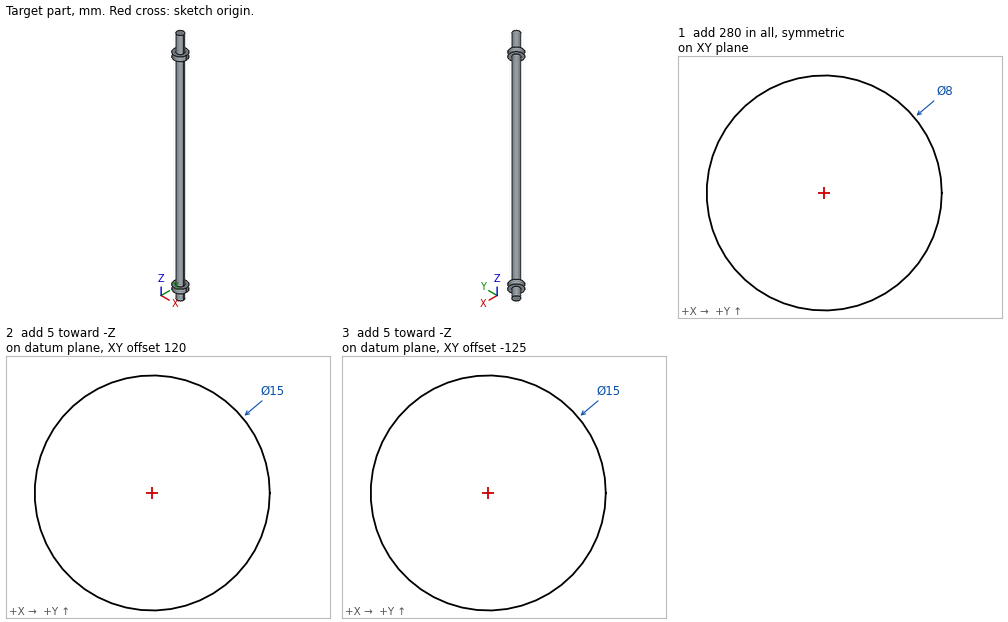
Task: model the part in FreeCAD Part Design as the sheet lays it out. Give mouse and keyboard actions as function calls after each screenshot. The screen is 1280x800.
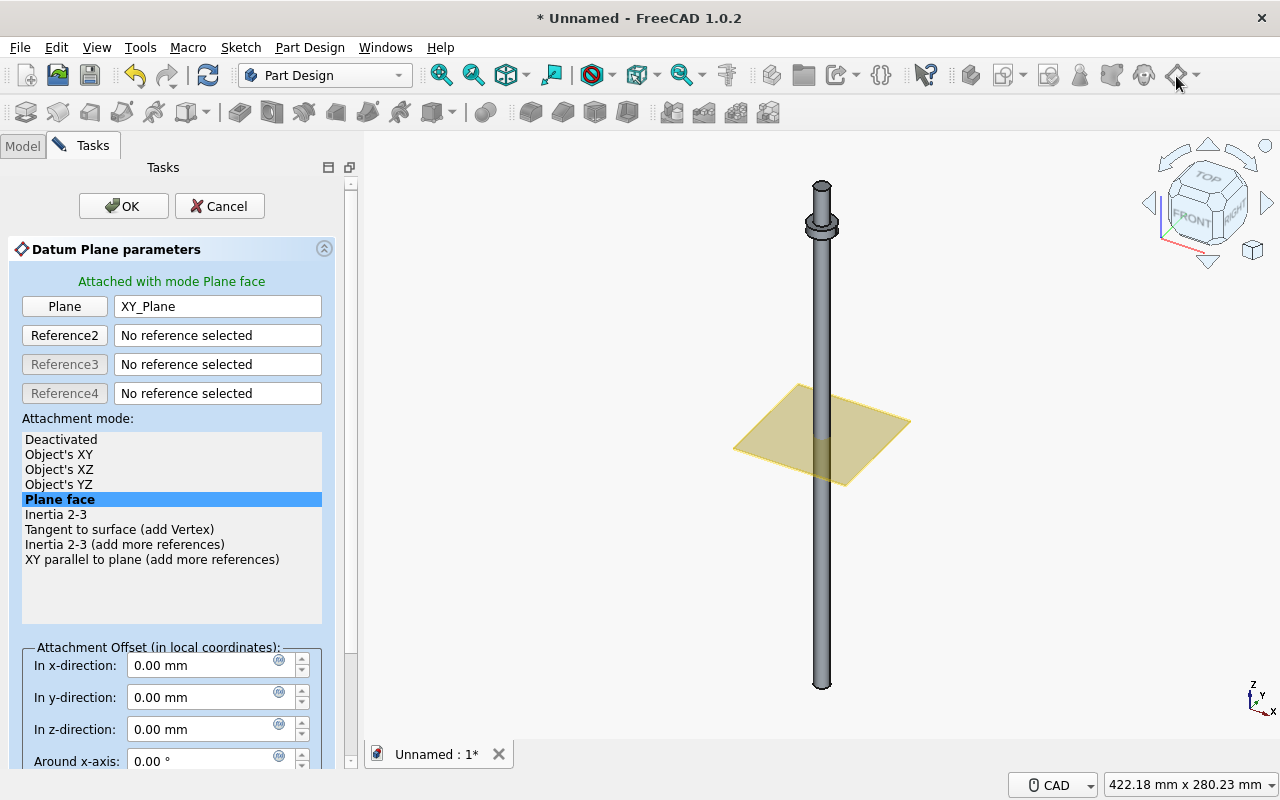
triple_click(210, 729)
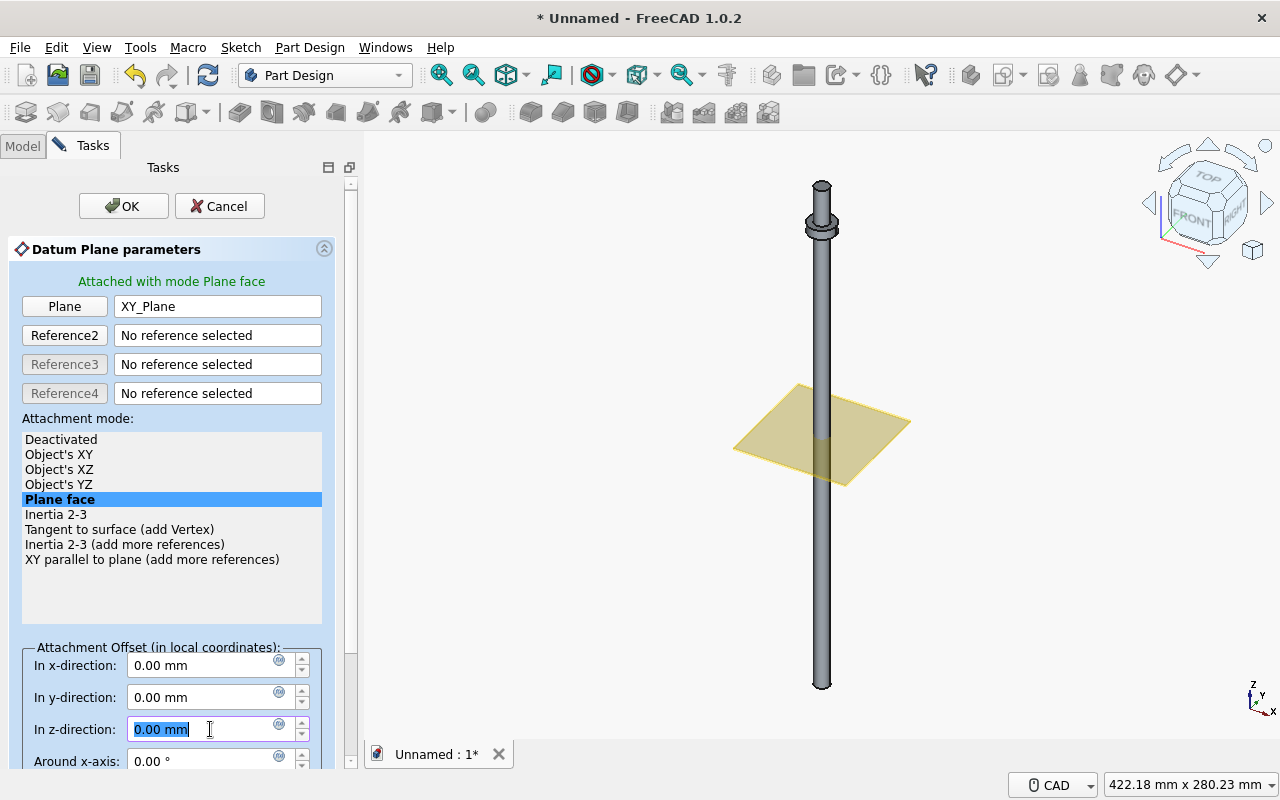
text(-125)
key(Tab)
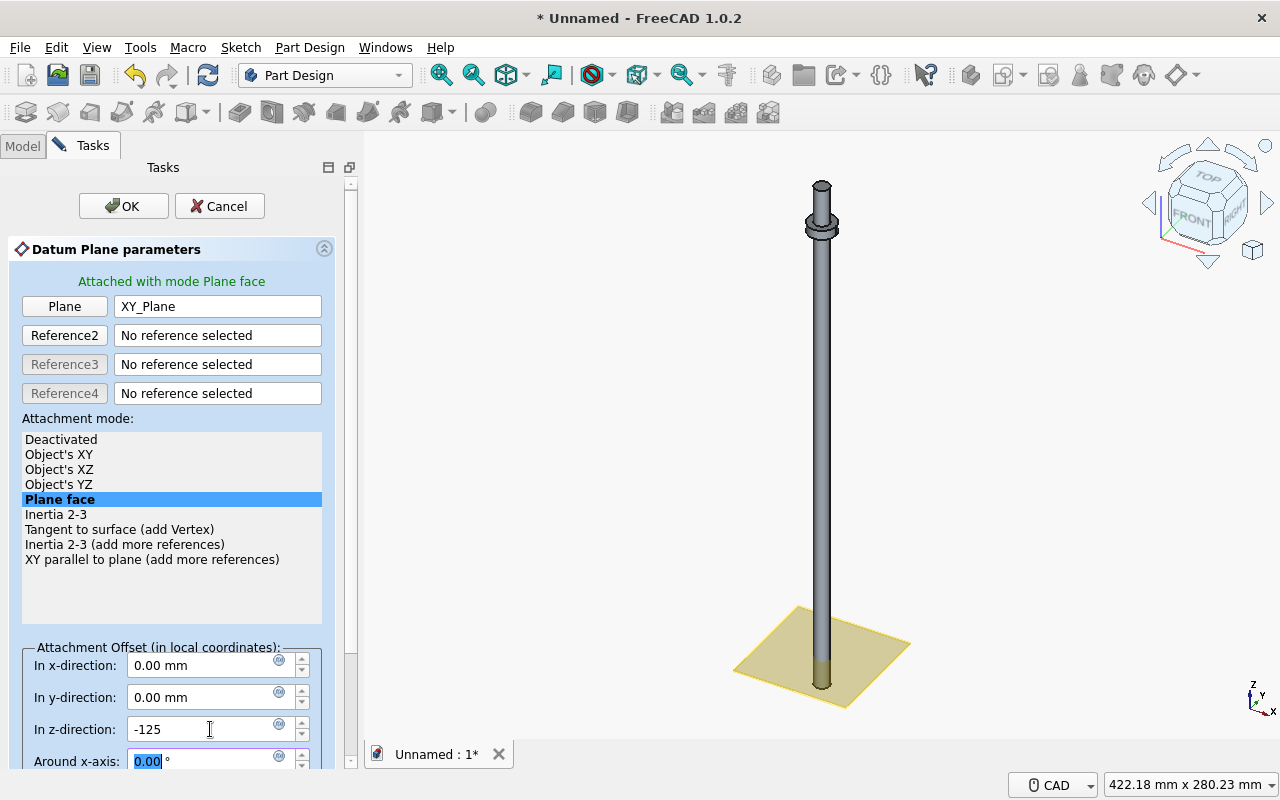
click(124, 206)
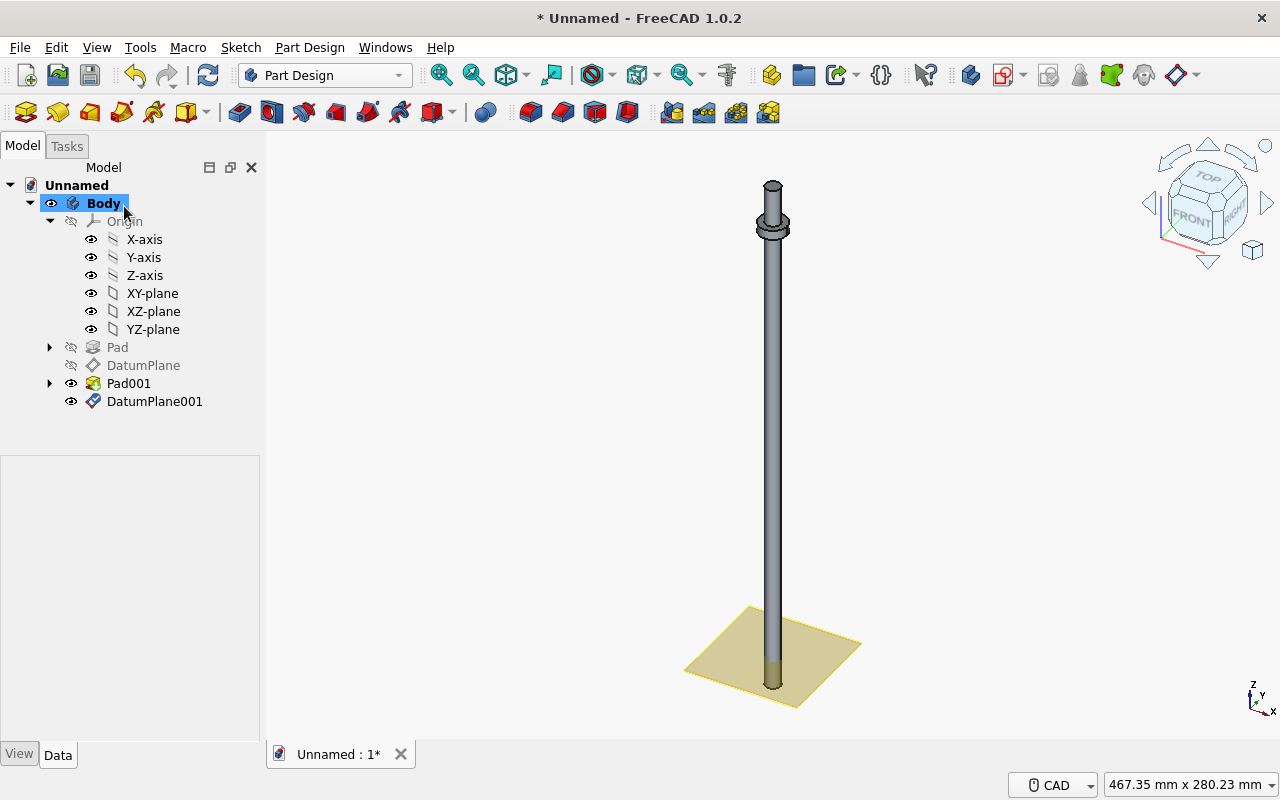
click(116, 401)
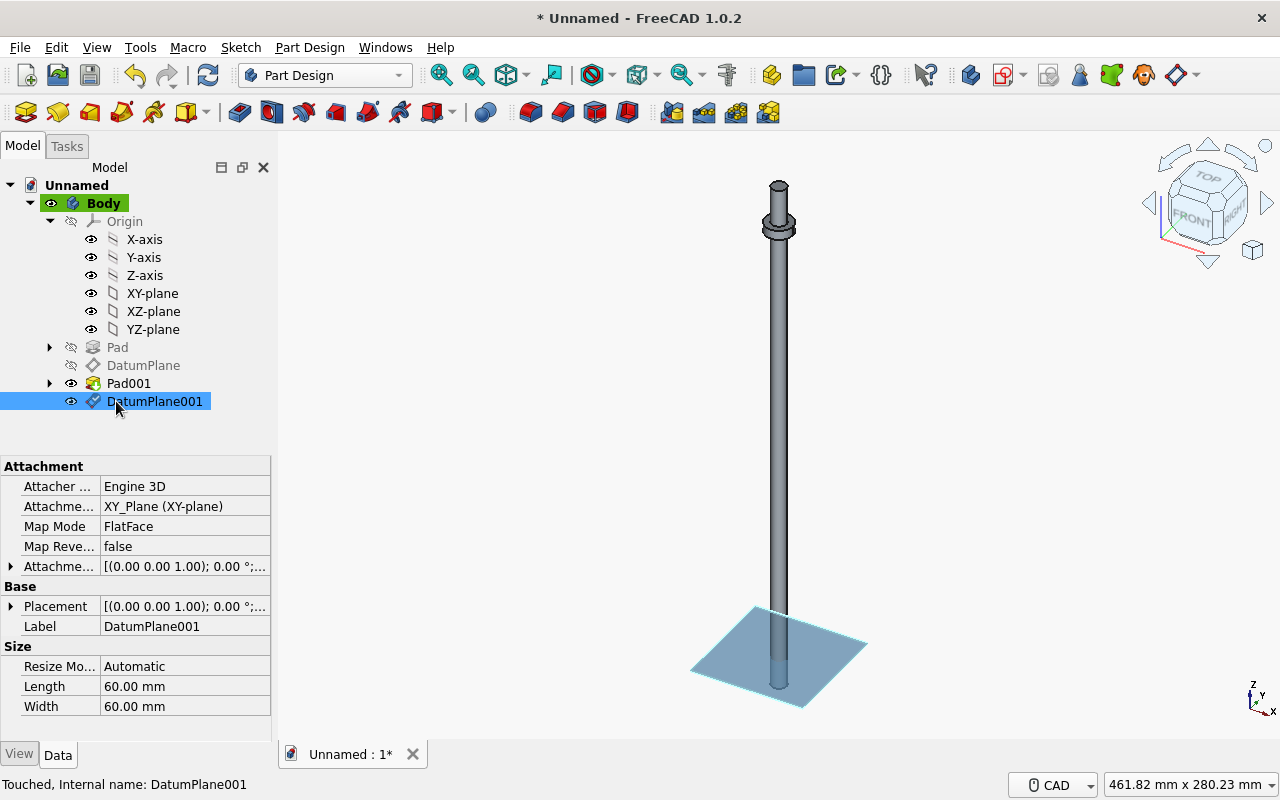
click(1004, 76)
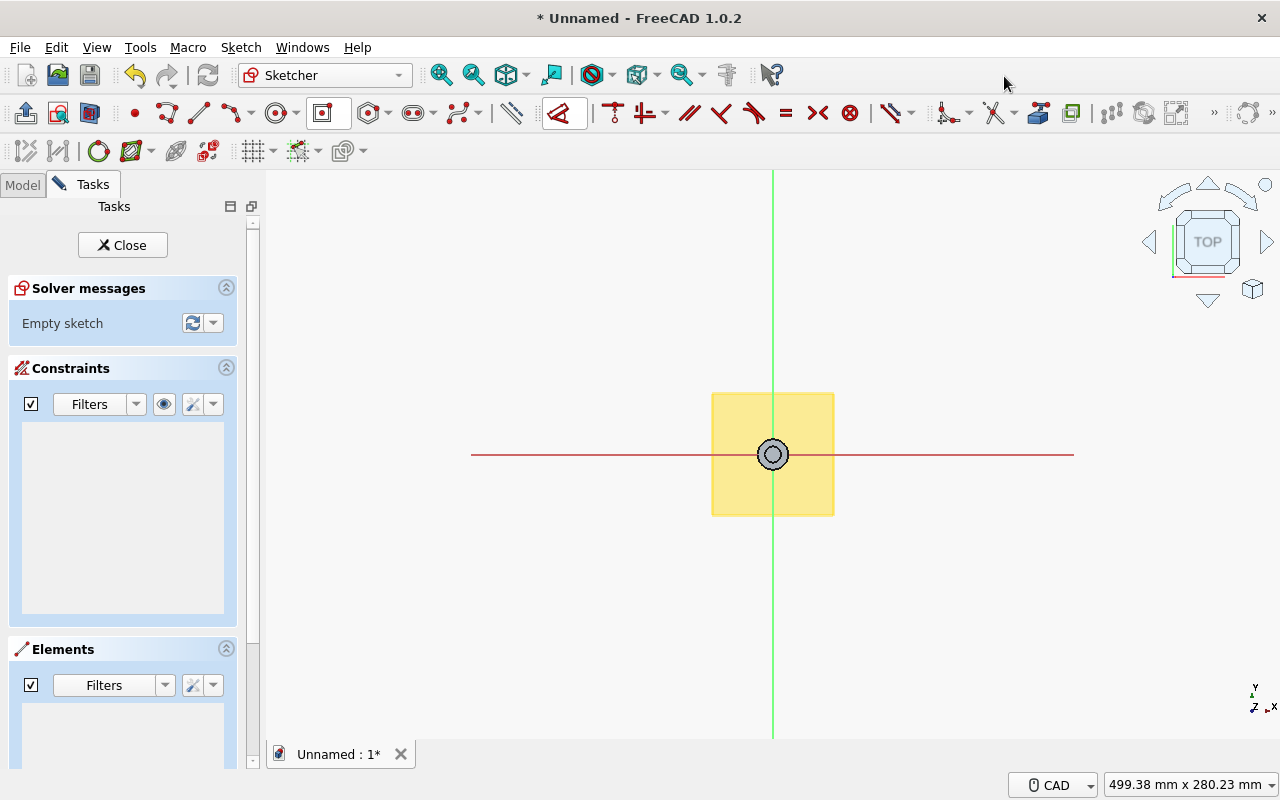
key(q)
key(s)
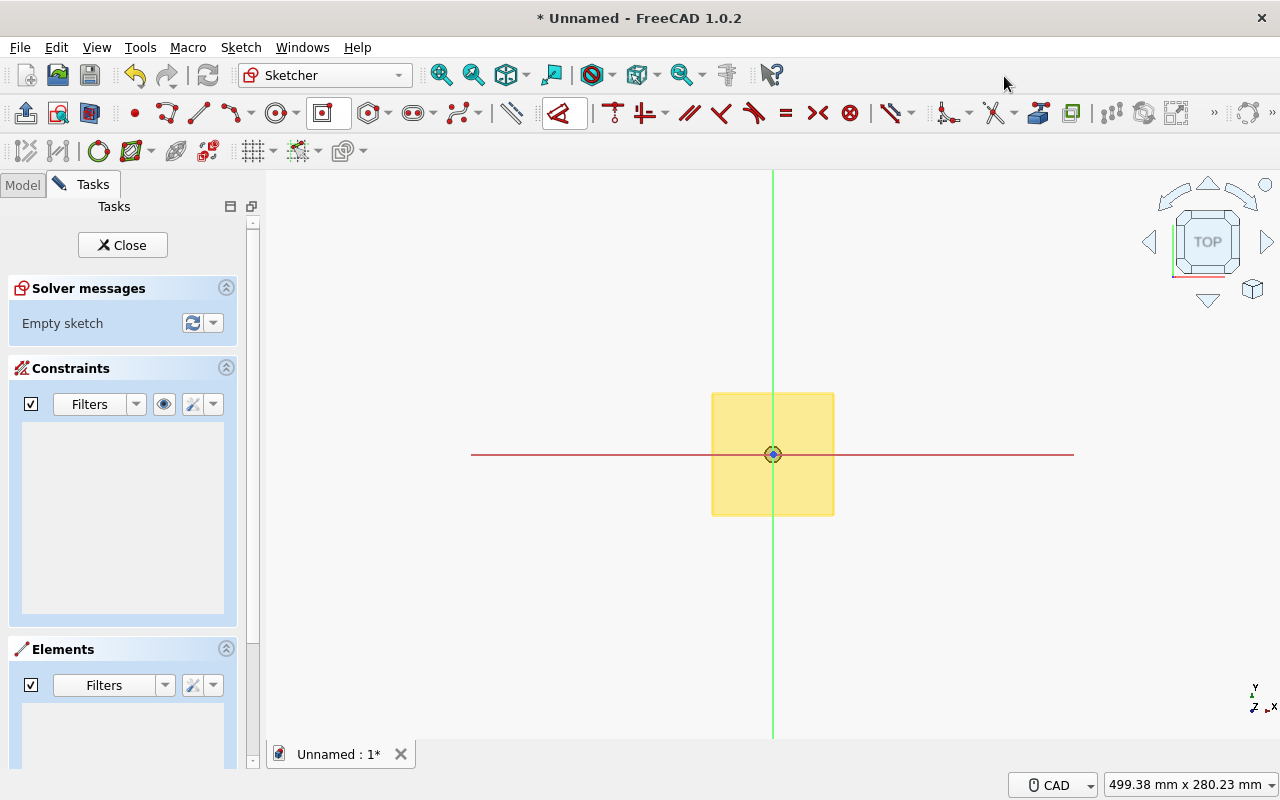
scroll(780, 455, up, 12)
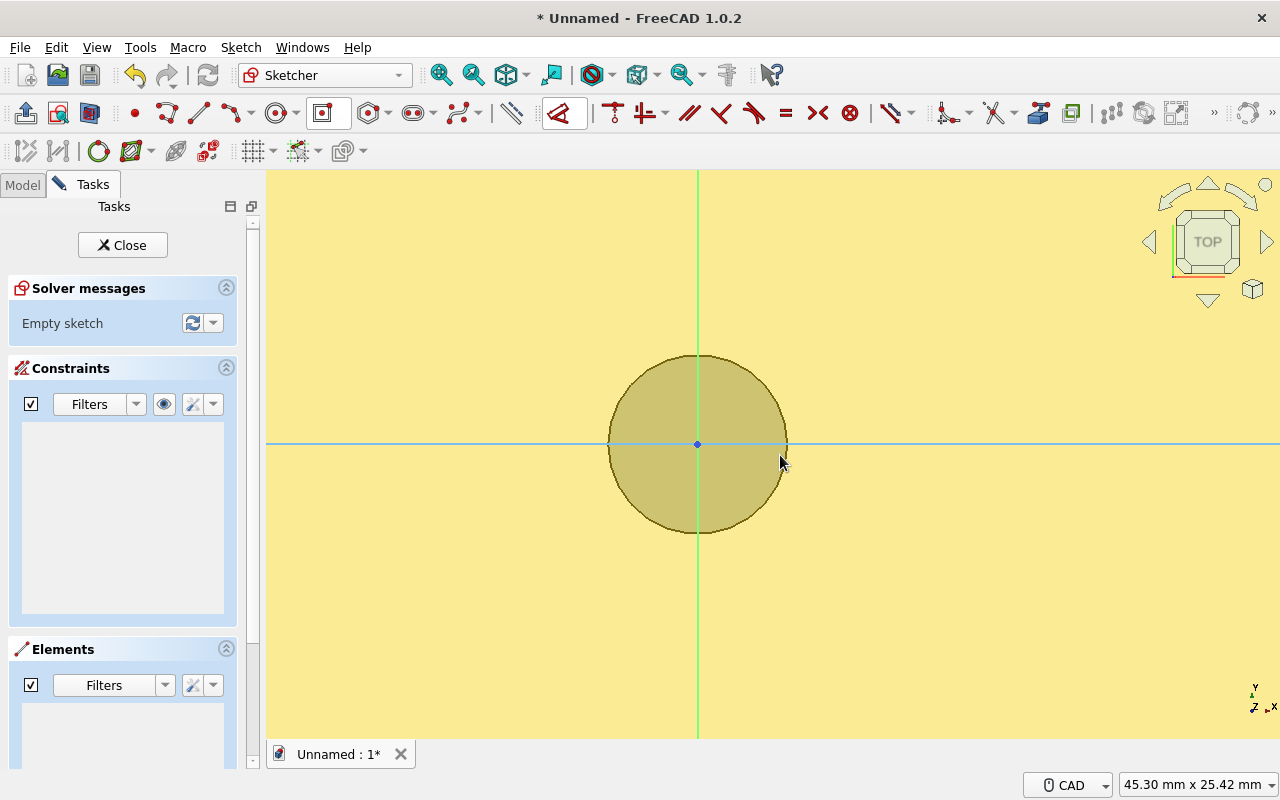
key(g)
key(c)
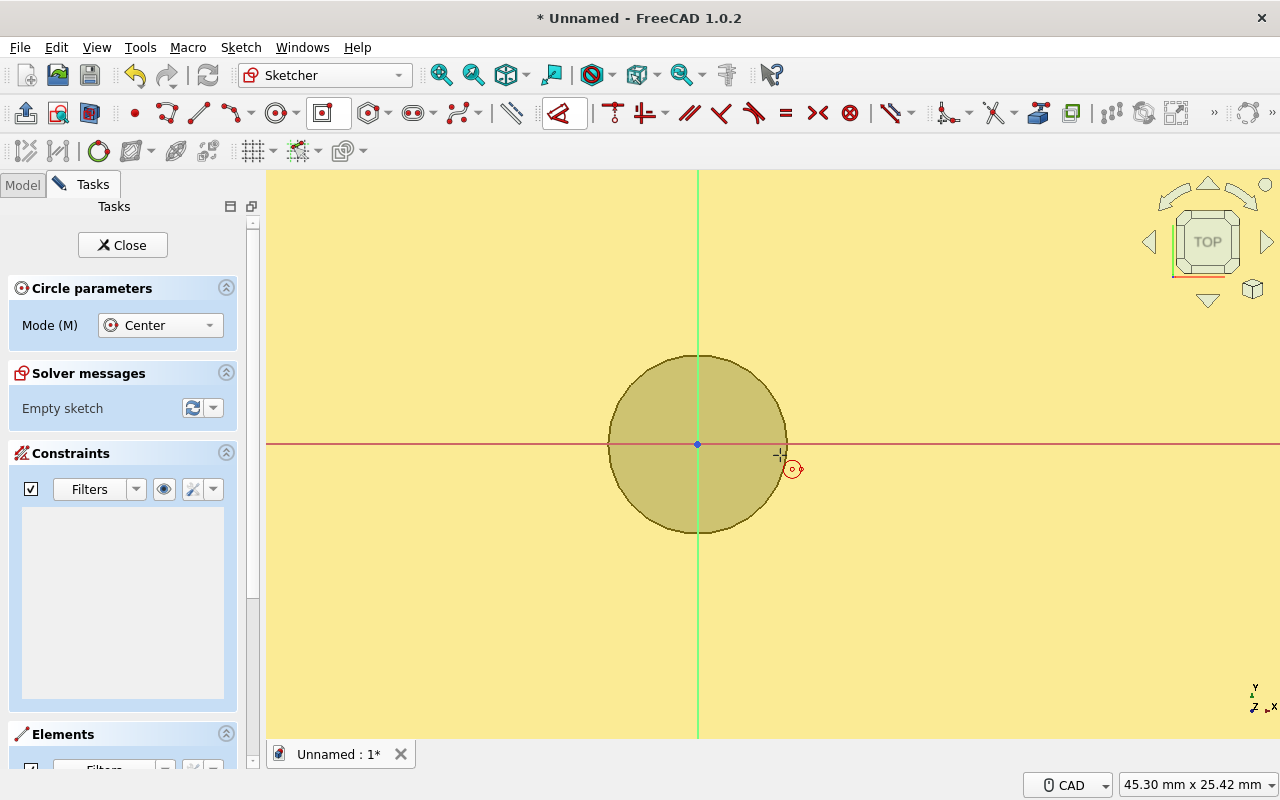
click(698, 444)
click(816, 326)
key(Escape)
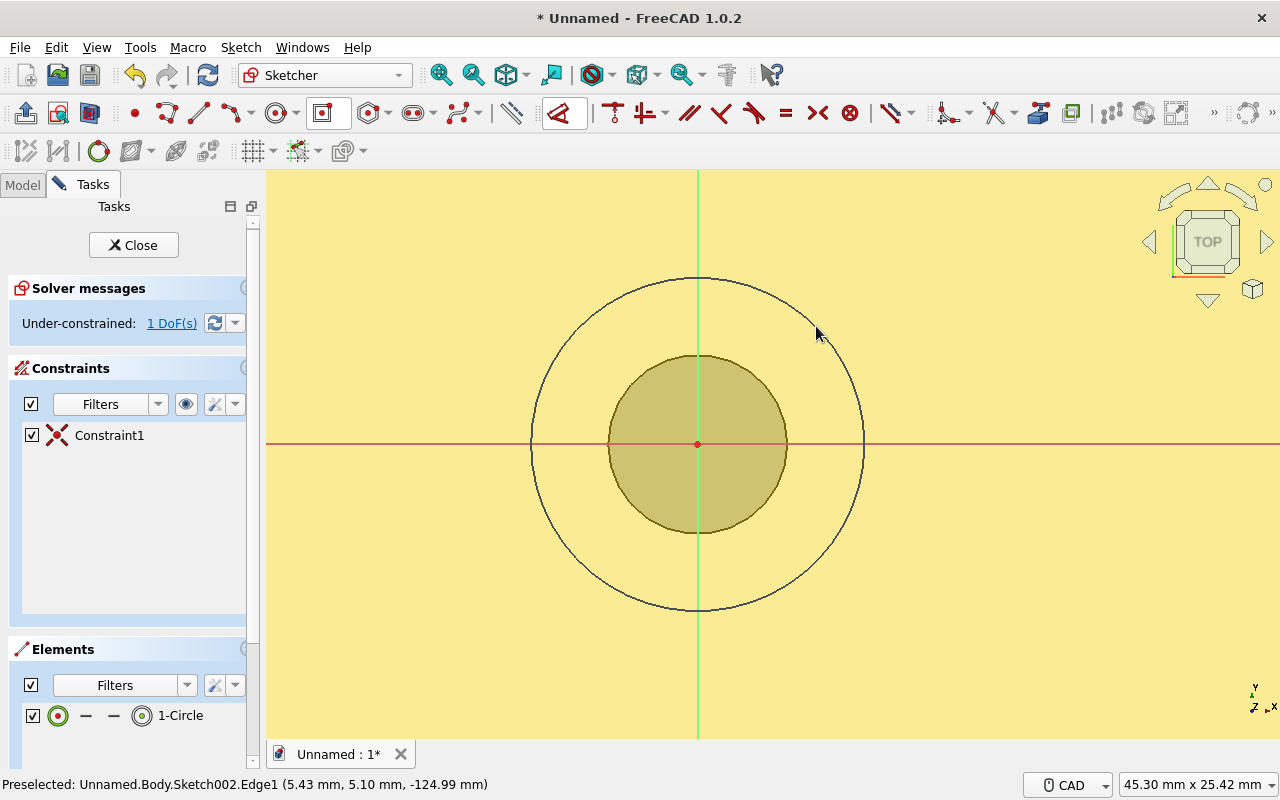
click(815, 326)